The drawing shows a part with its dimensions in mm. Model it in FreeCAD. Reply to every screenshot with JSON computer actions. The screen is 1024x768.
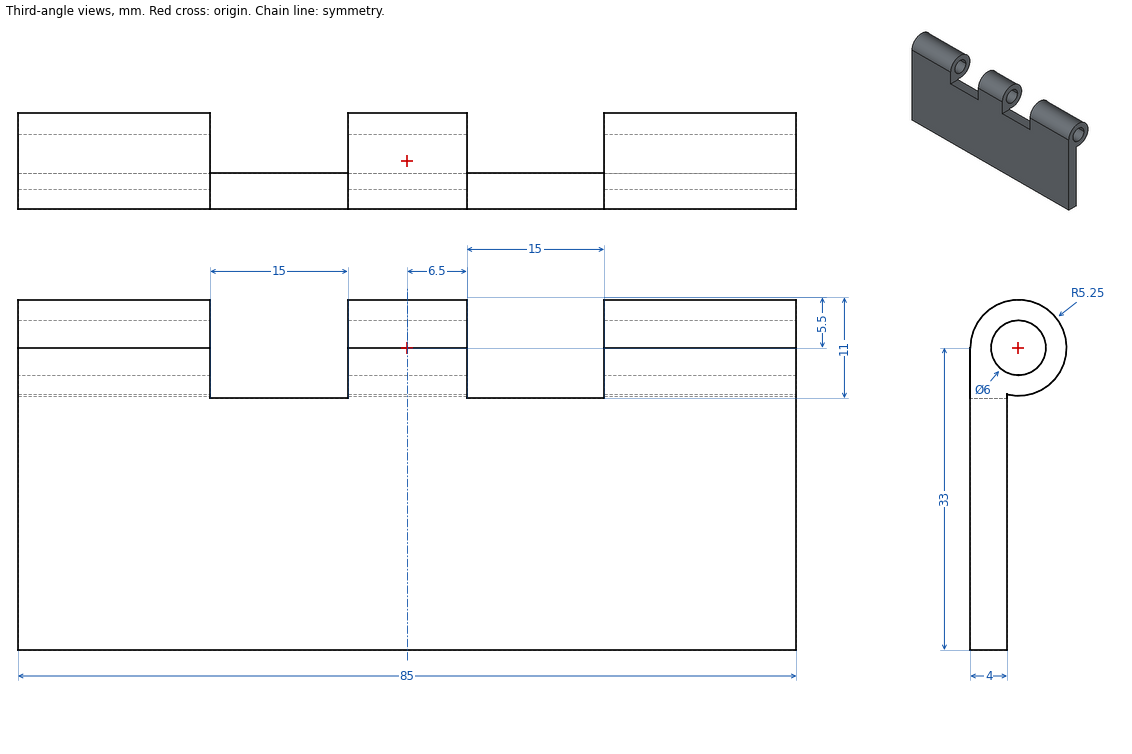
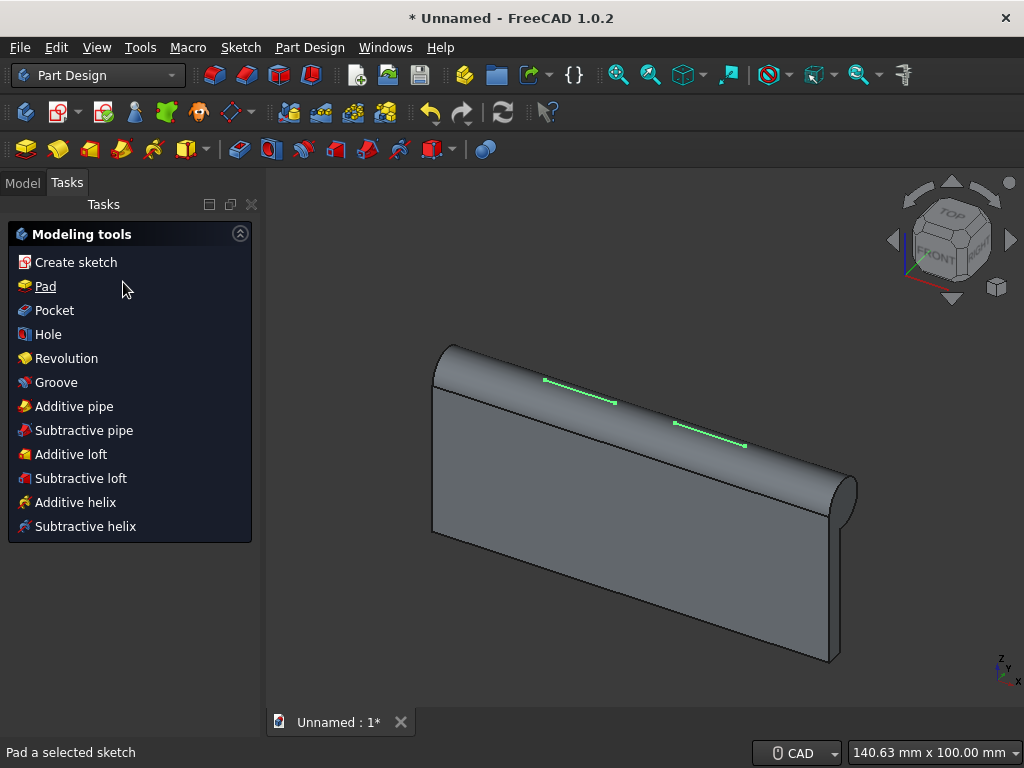
{"action": "left_click", "coordinate": [240, 150]}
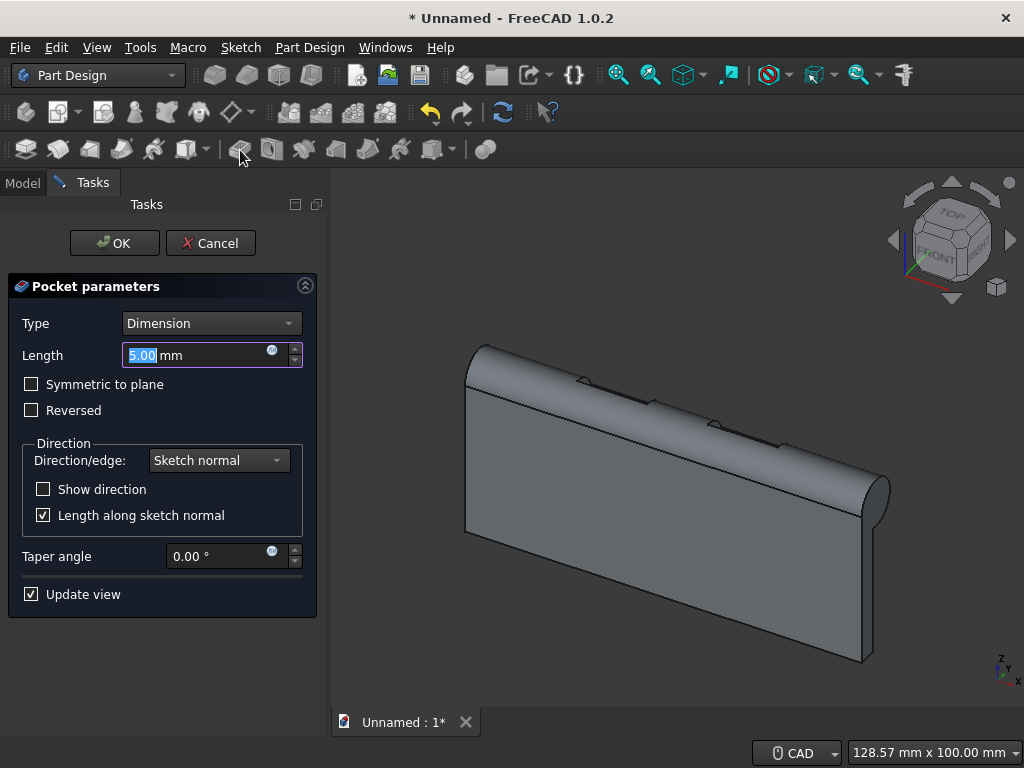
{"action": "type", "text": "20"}
{"action": "key", "text": "Tab"}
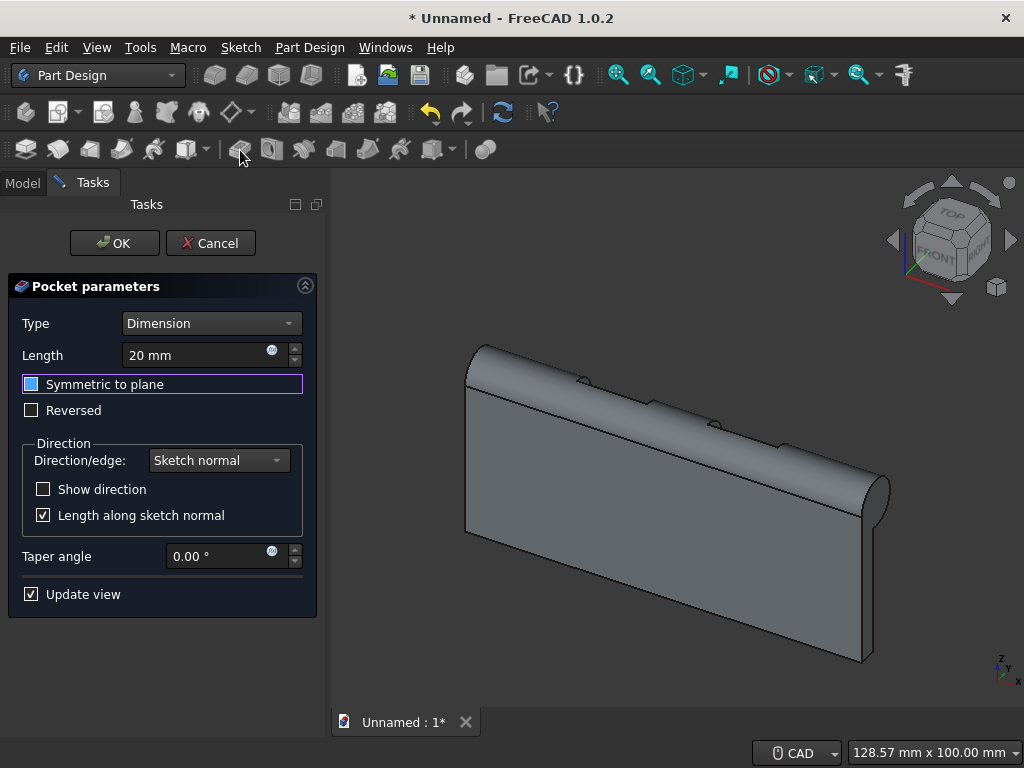
{"action": "left_click", "coordinate": [30, 384]}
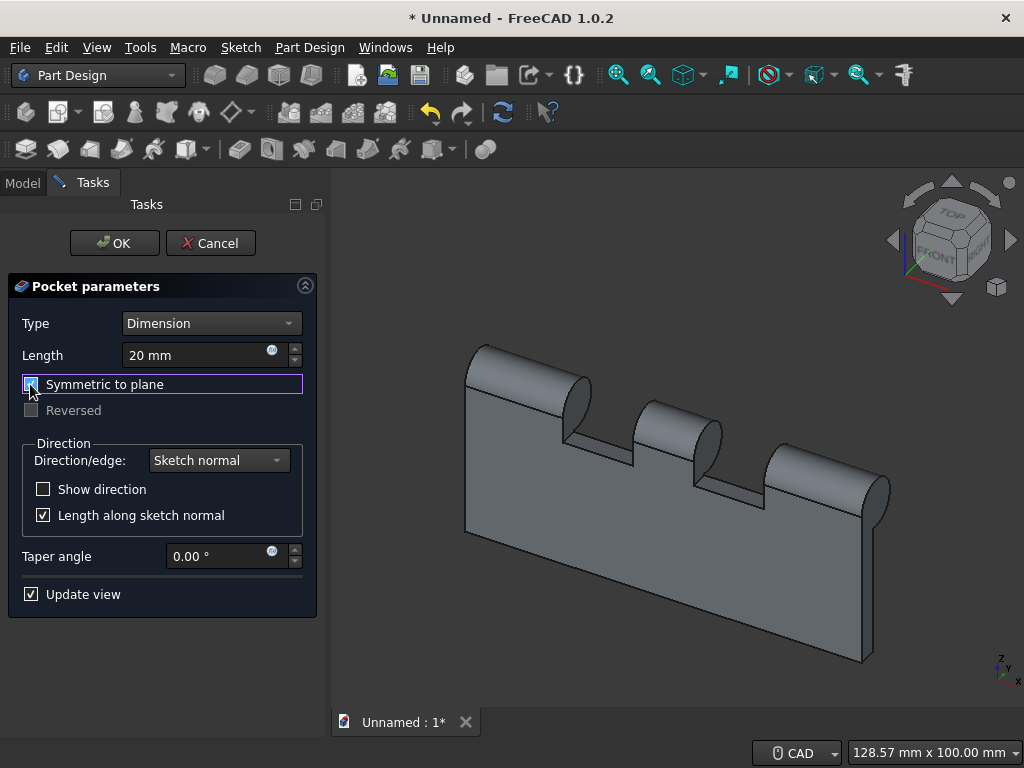
{"action": "left_click", "coordinate": [115, 243]}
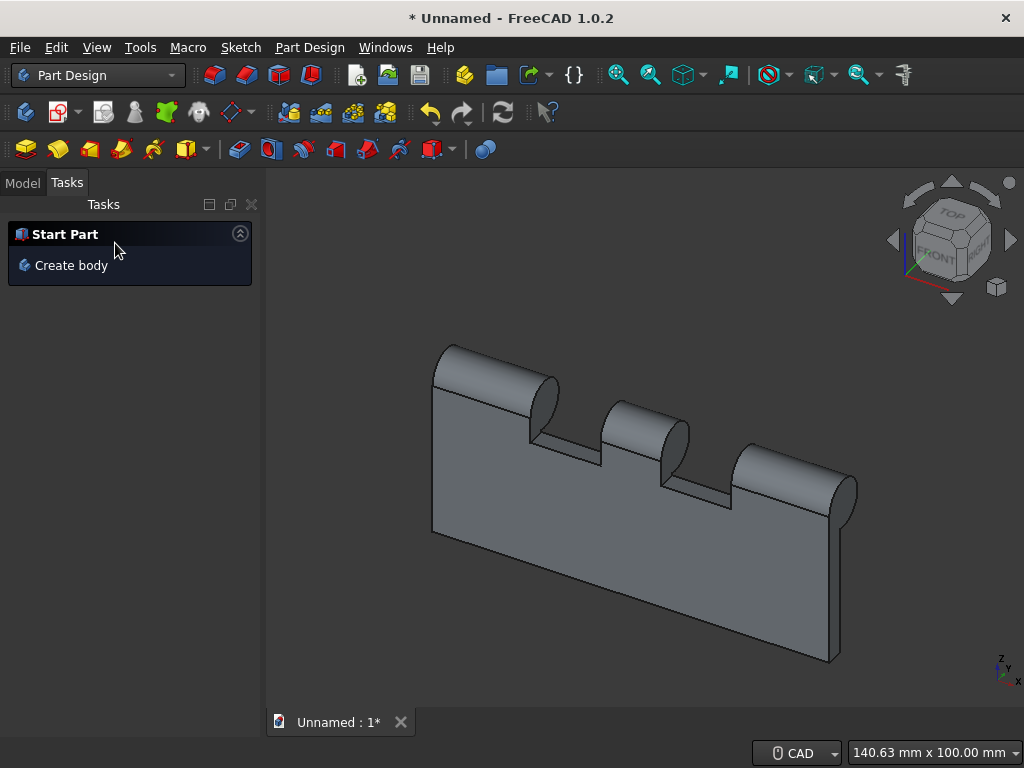
{"action": "left_click", "coordinate": [843, 515]}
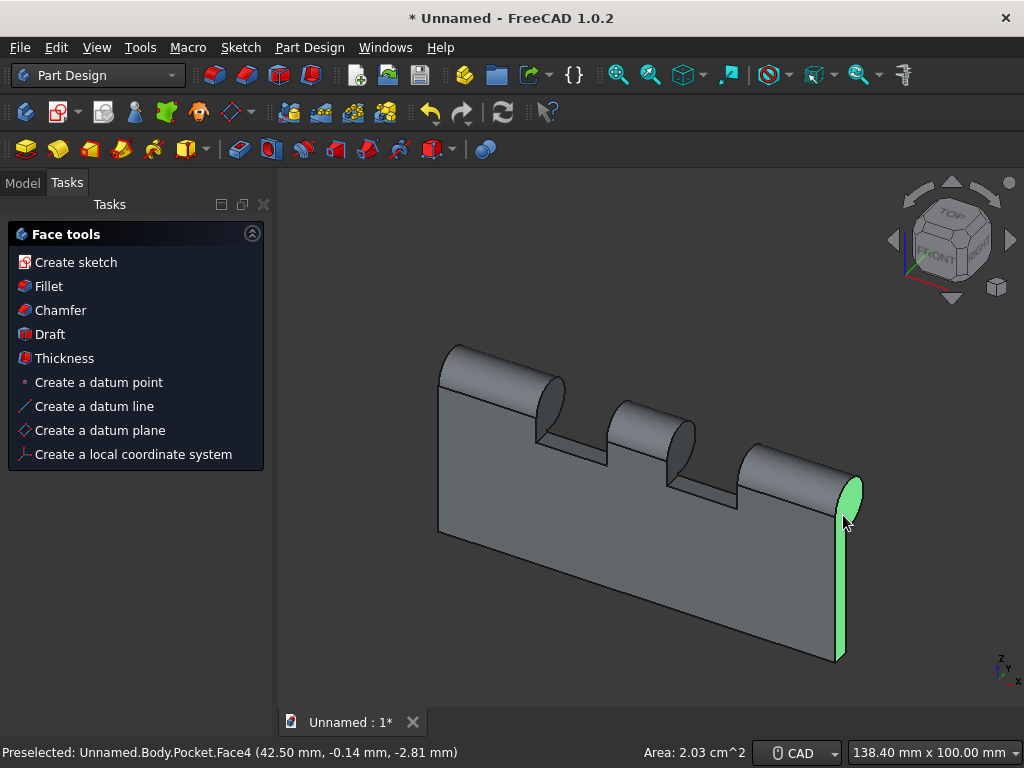
{"action": "left_click", "coordinate": [58, 112]}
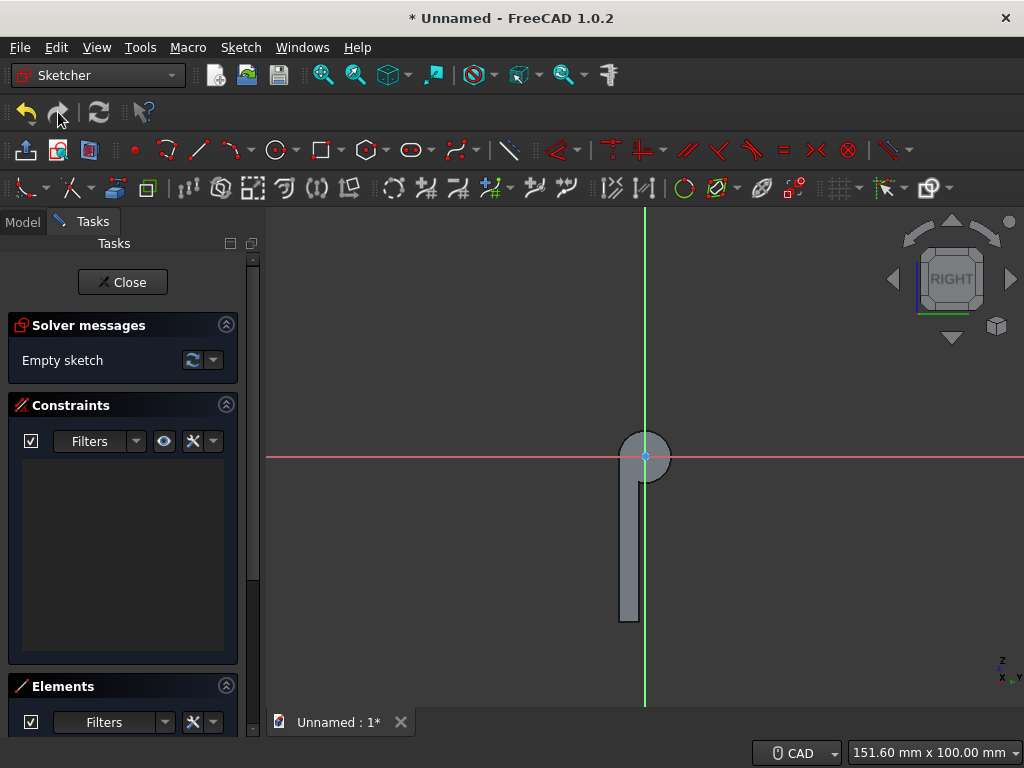
{"action": "scroll", "coordinate": [652, 457], "scroll_direction": "up", "scroll_amount": 12}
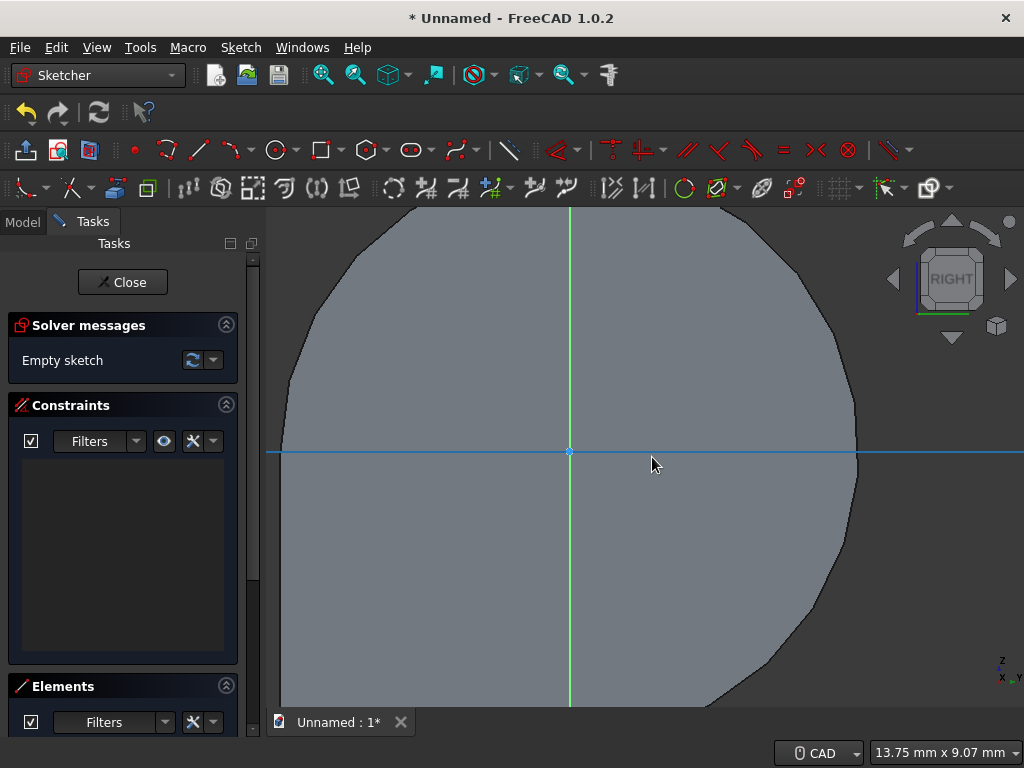
{"action": "left_click", "coordinate": [276, 150]}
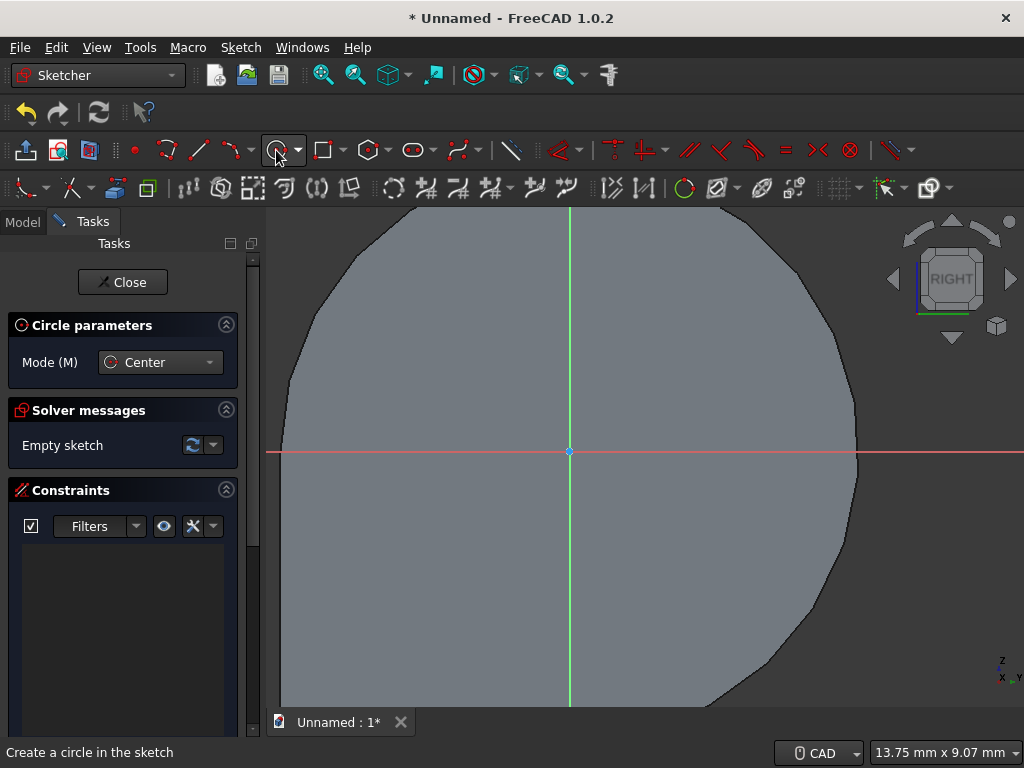
{"action": "left_click", "coordinate": [570, 452]}
{"action": "mouse_move", "coordinate": [687, 335]}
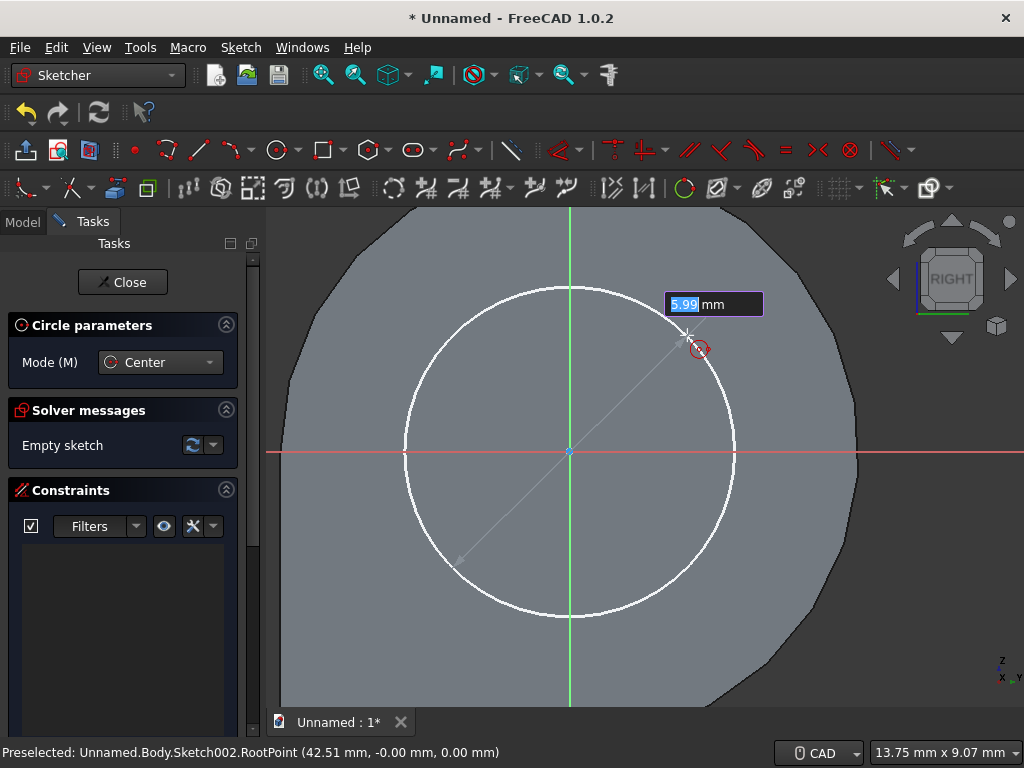
{"action": "type", "text": "6"}
{"action": "key", "text": "Return"}
{"action": "key", "text": "Escape"}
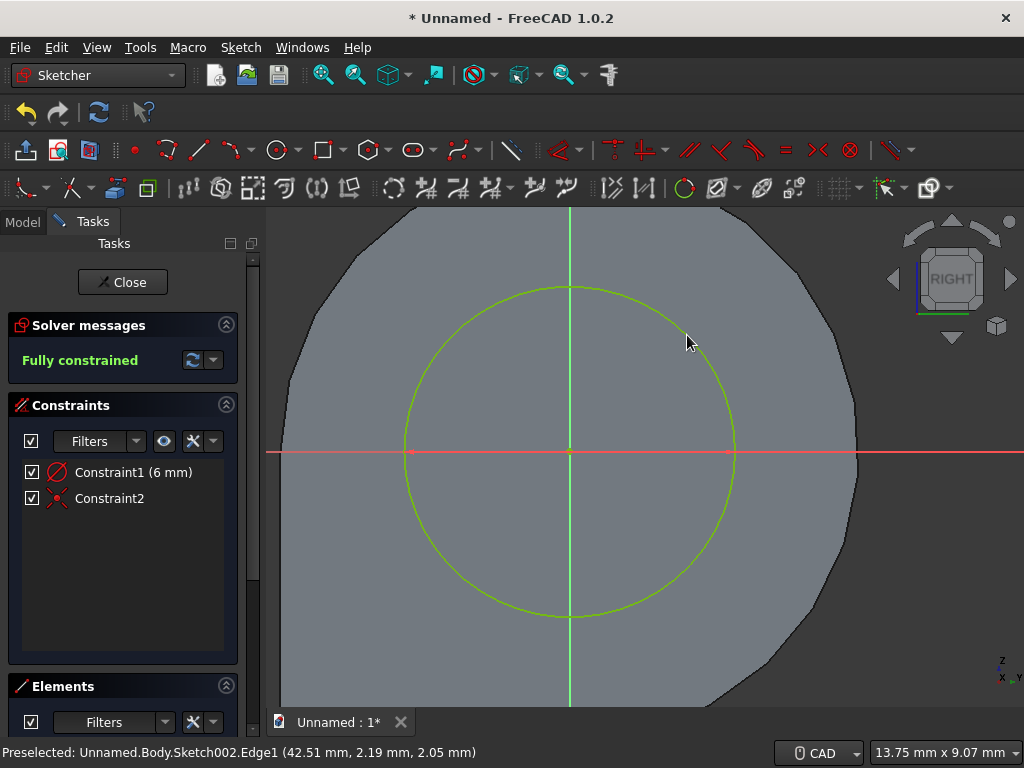
{"action": "left_click", "coordinate": [123, 282]}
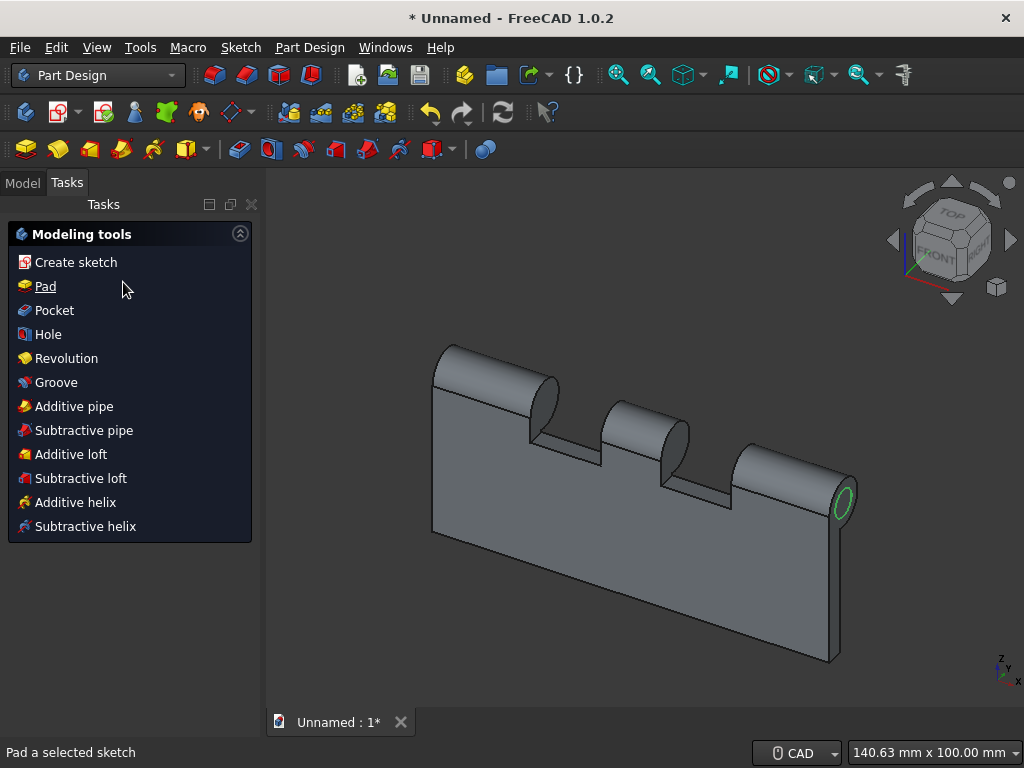
{"action": "left_click", "coordinate": [240, 150]}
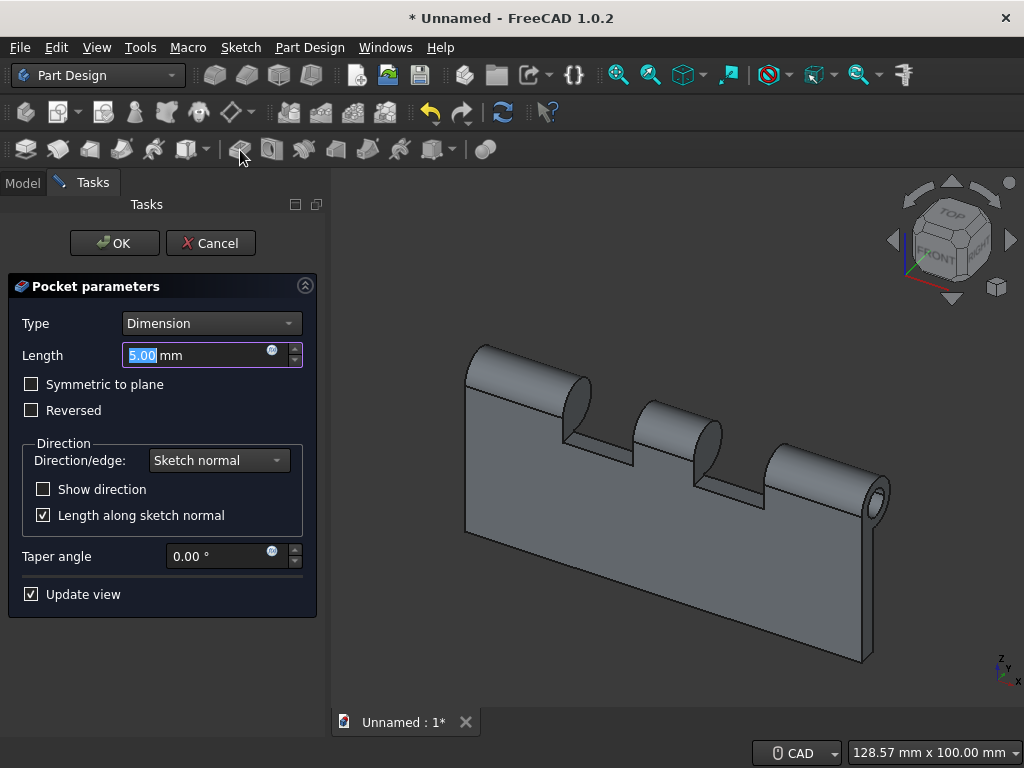
{"action": "left_click", "coordinate": [212, 324]}